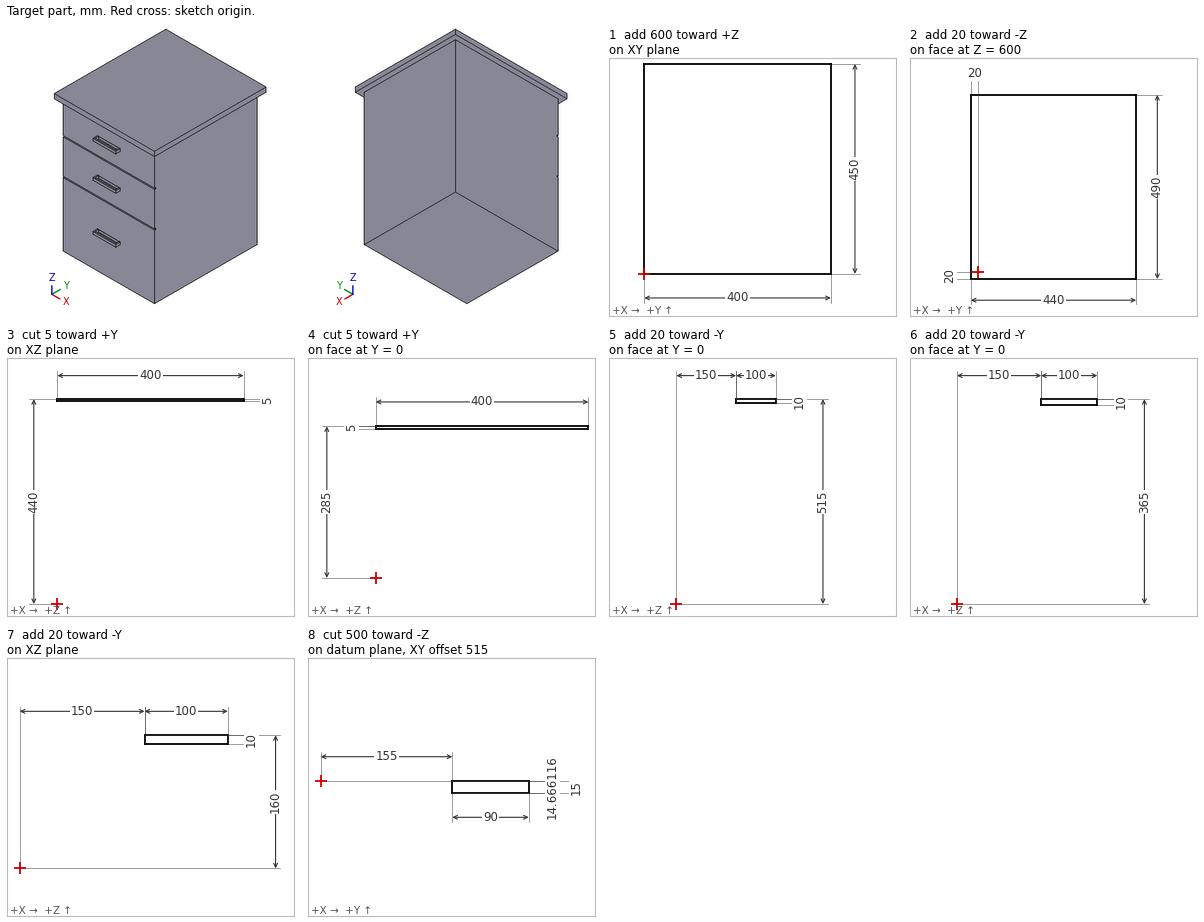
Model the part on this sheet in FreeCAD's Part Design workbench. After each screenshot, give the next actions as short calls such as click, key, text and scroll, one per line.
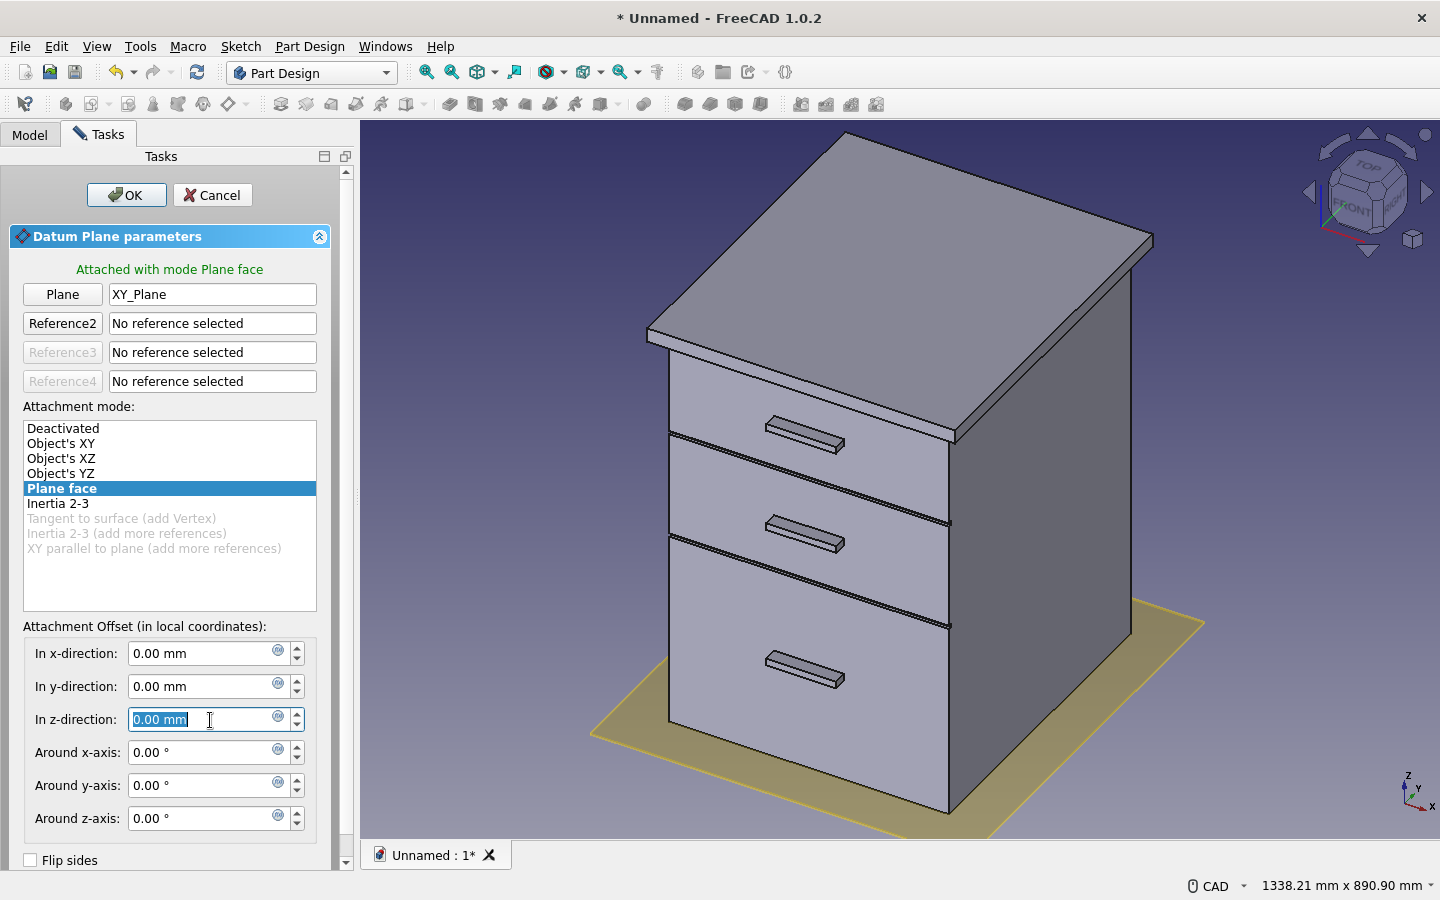
text(515)
key(Tab)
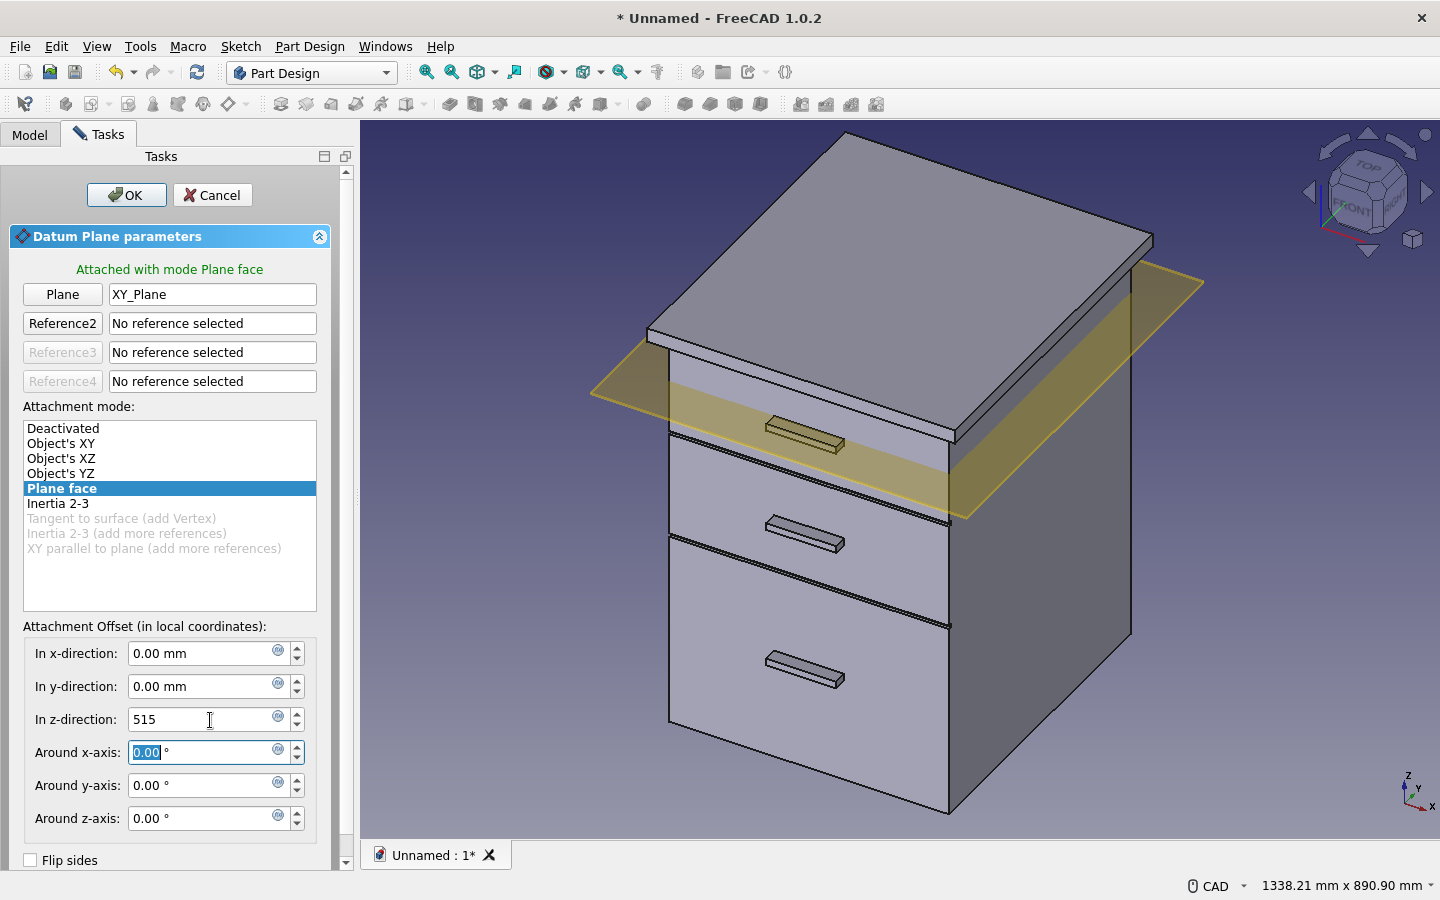
click(127, 195)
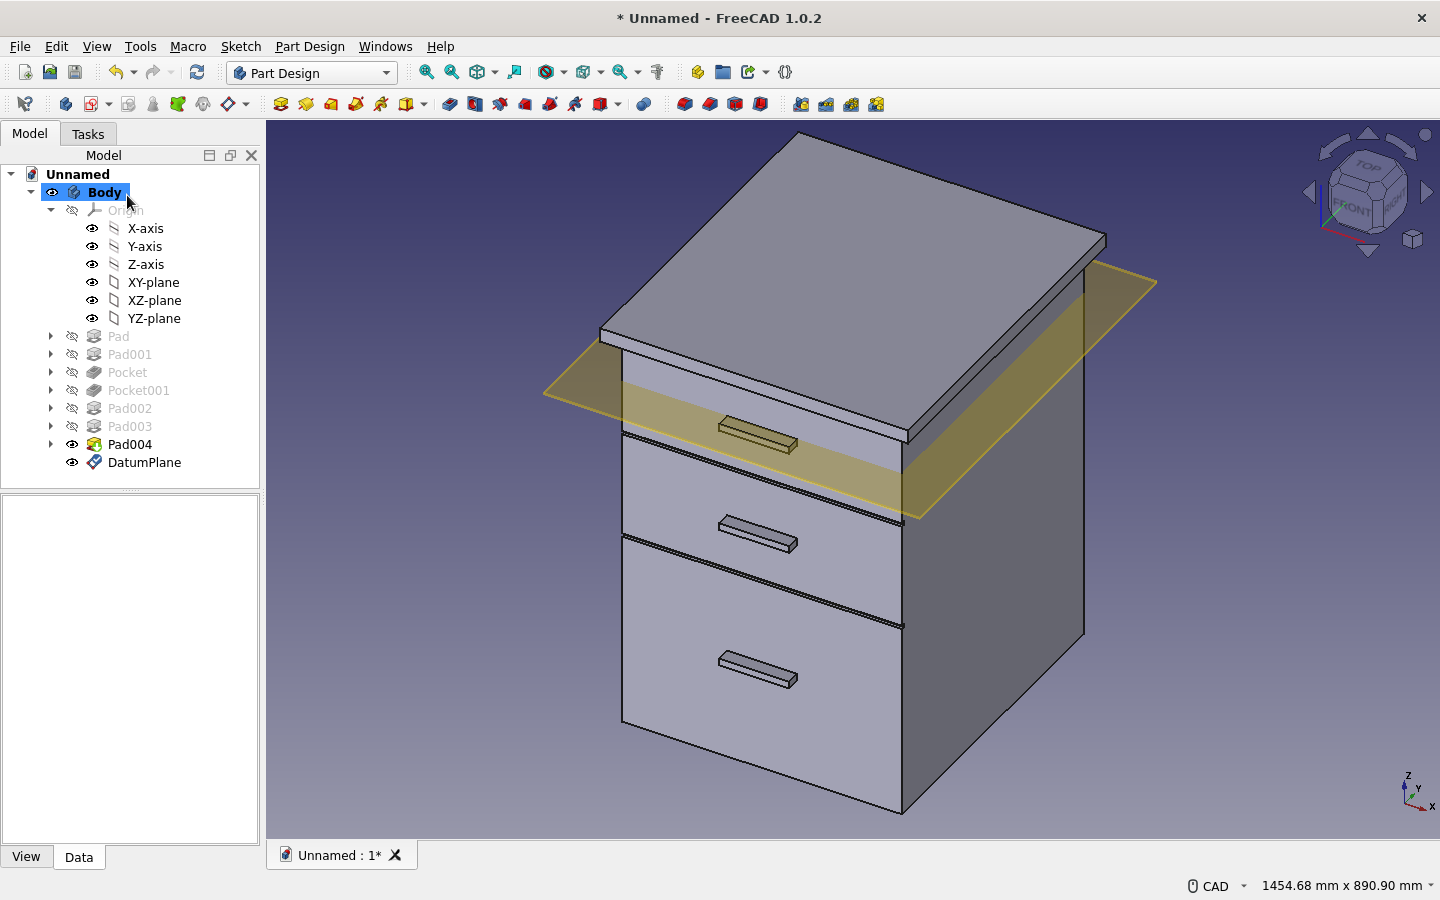
click(117, 462)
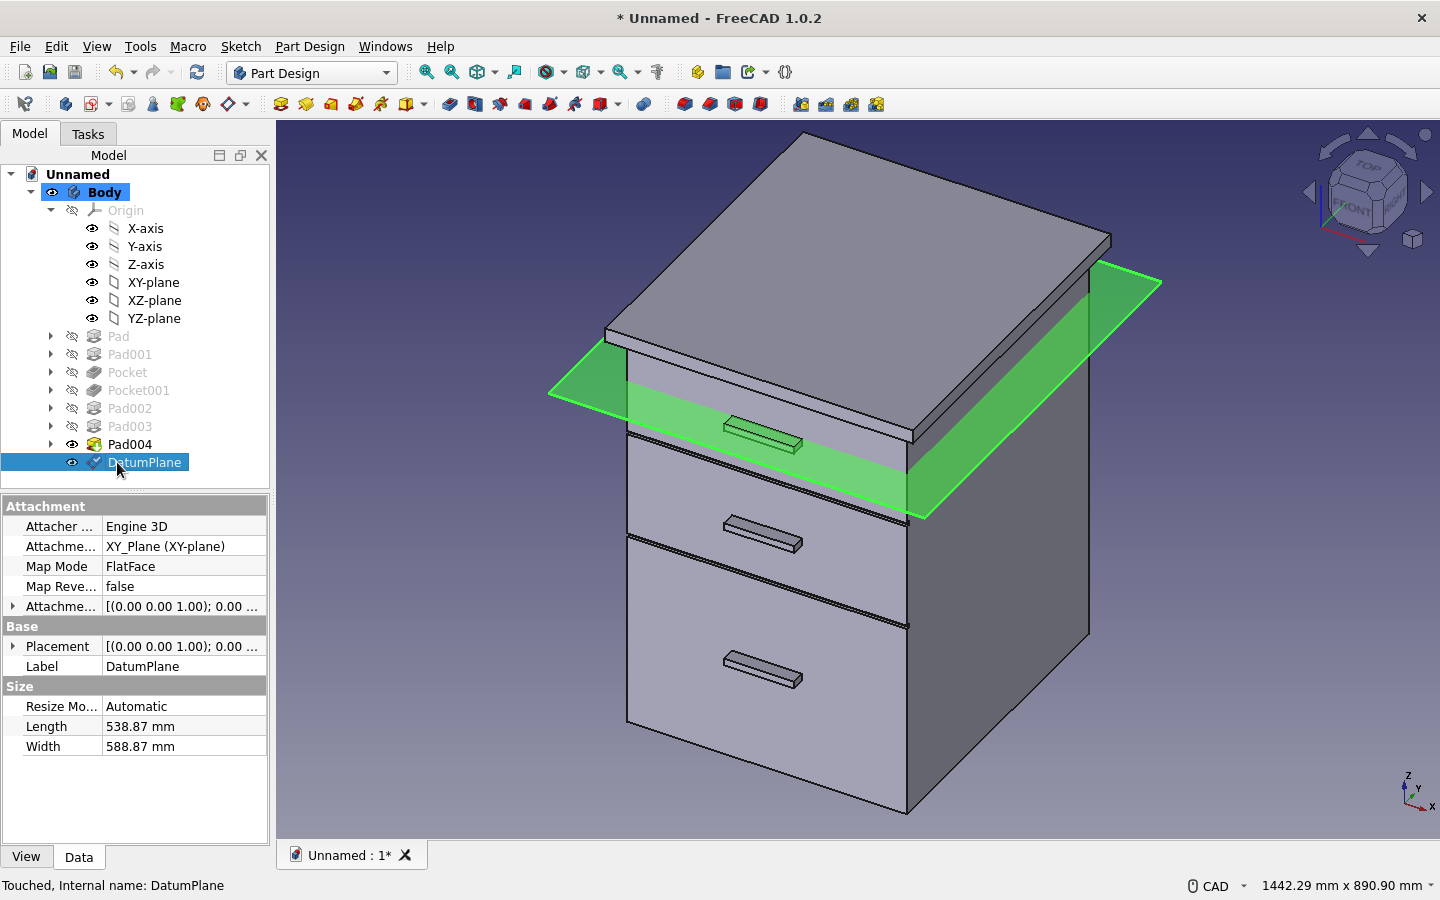
click(90, 104)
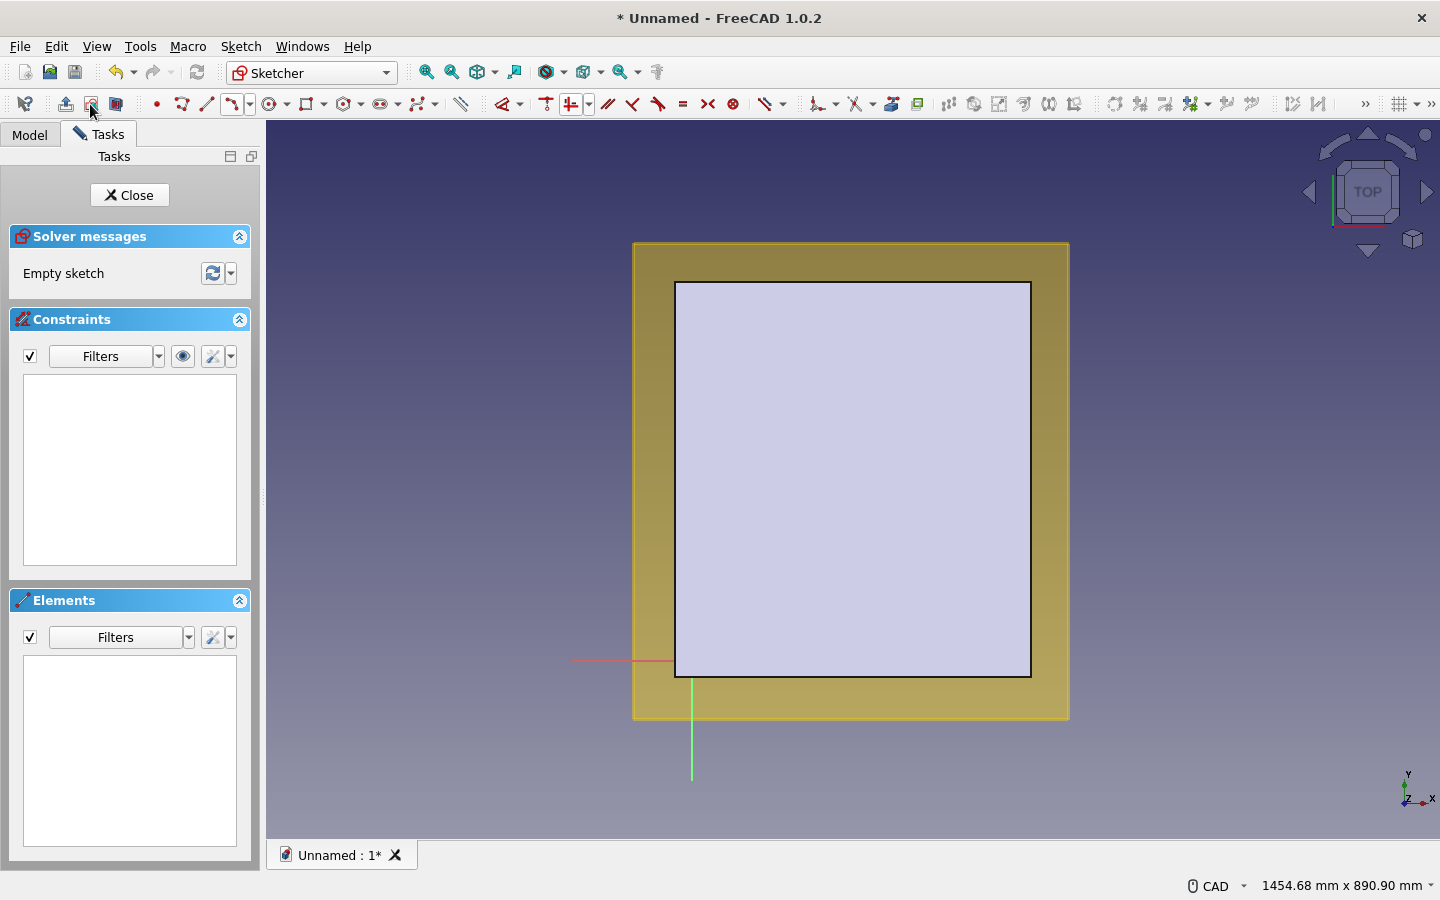
click(116, 104)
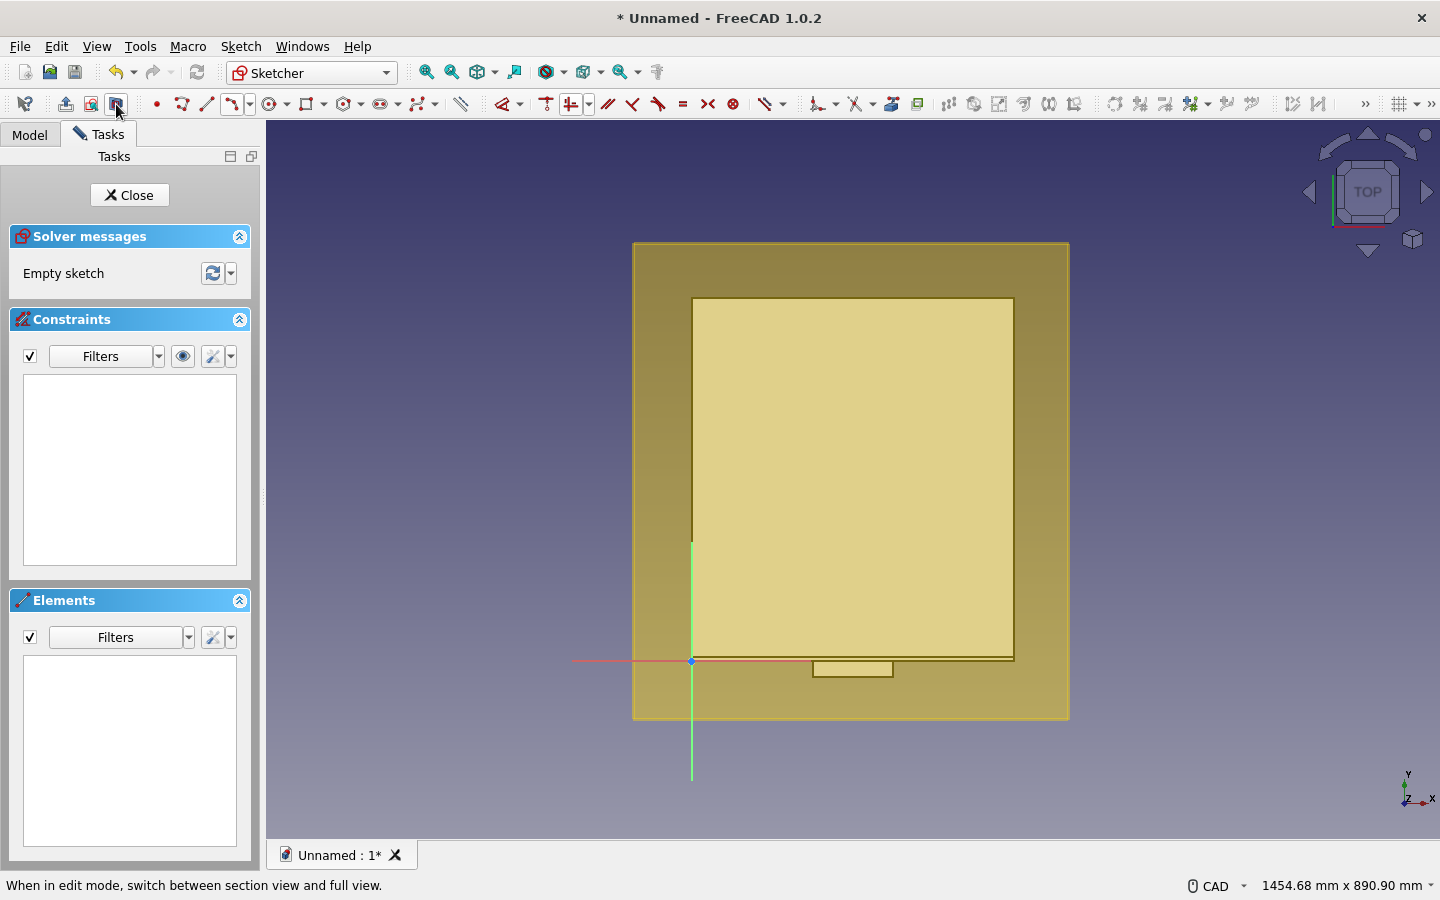
scroll(862, 691, up, 11)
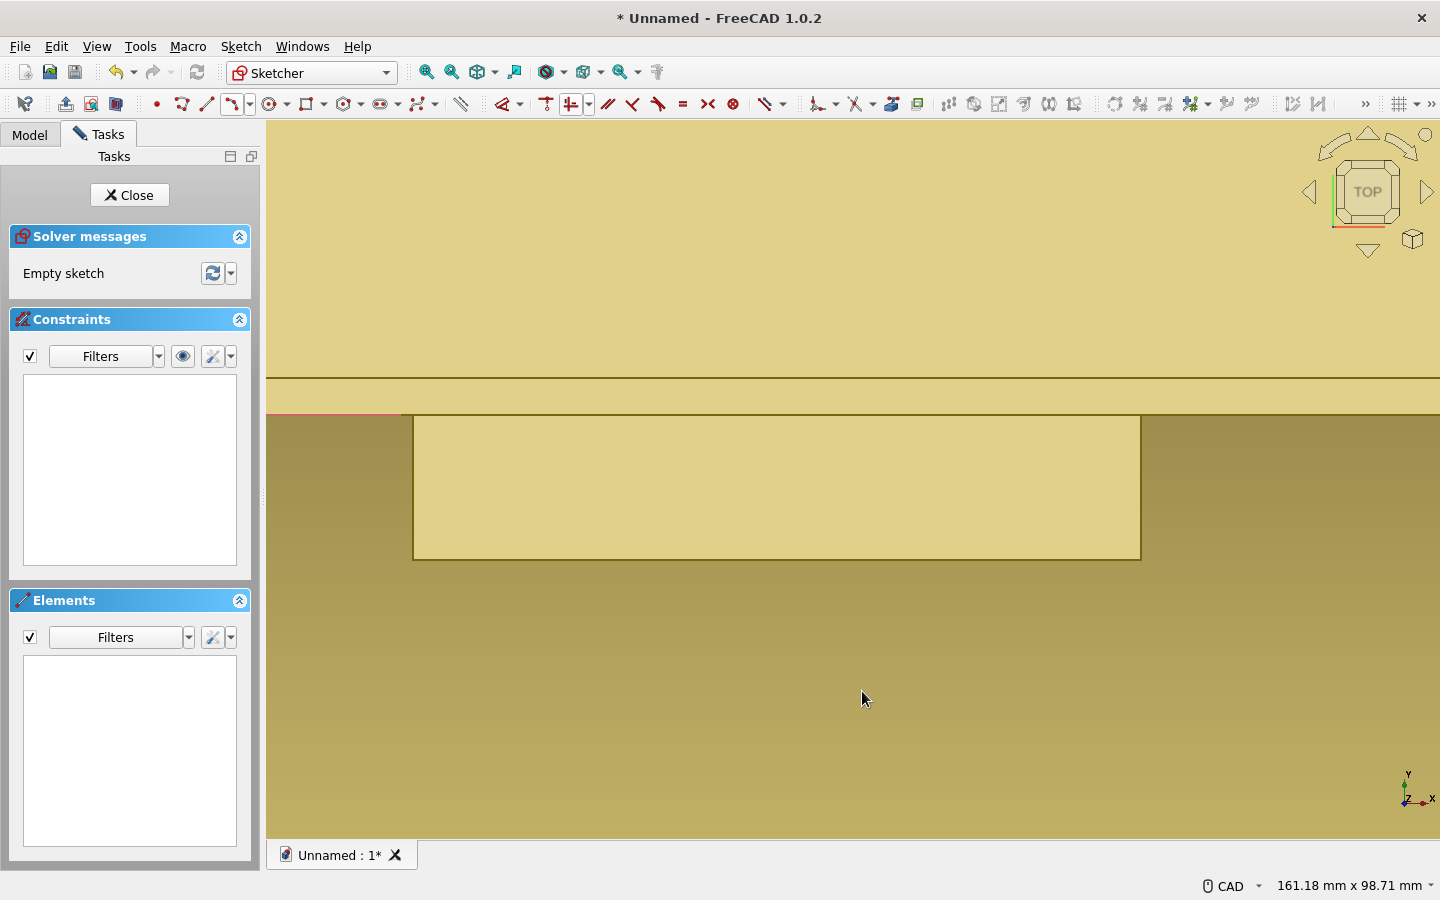
click(306, 104)